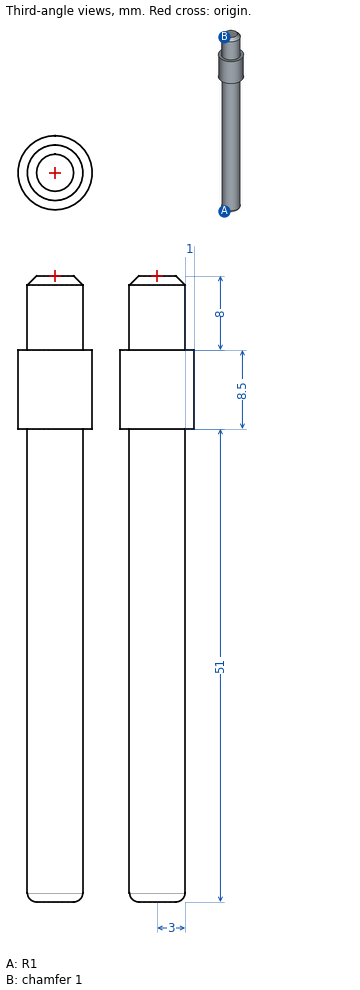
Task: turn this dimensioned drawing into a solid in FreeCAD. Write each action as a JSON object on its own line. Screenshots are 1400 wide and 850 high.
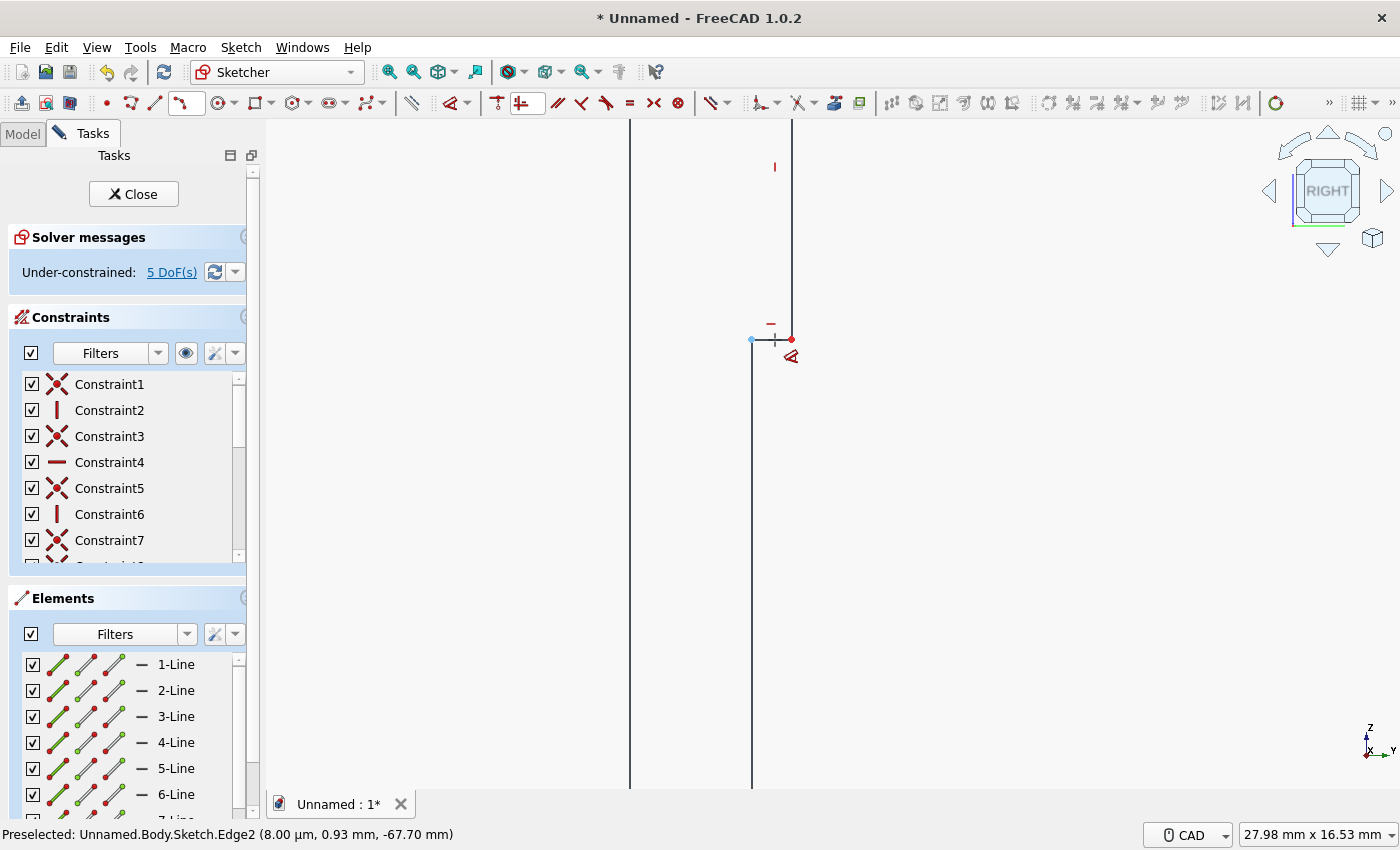
{"action": "left_click", "coordinate": [772, 340]}
{"action": "left_click", "coordinate": [772, 306]}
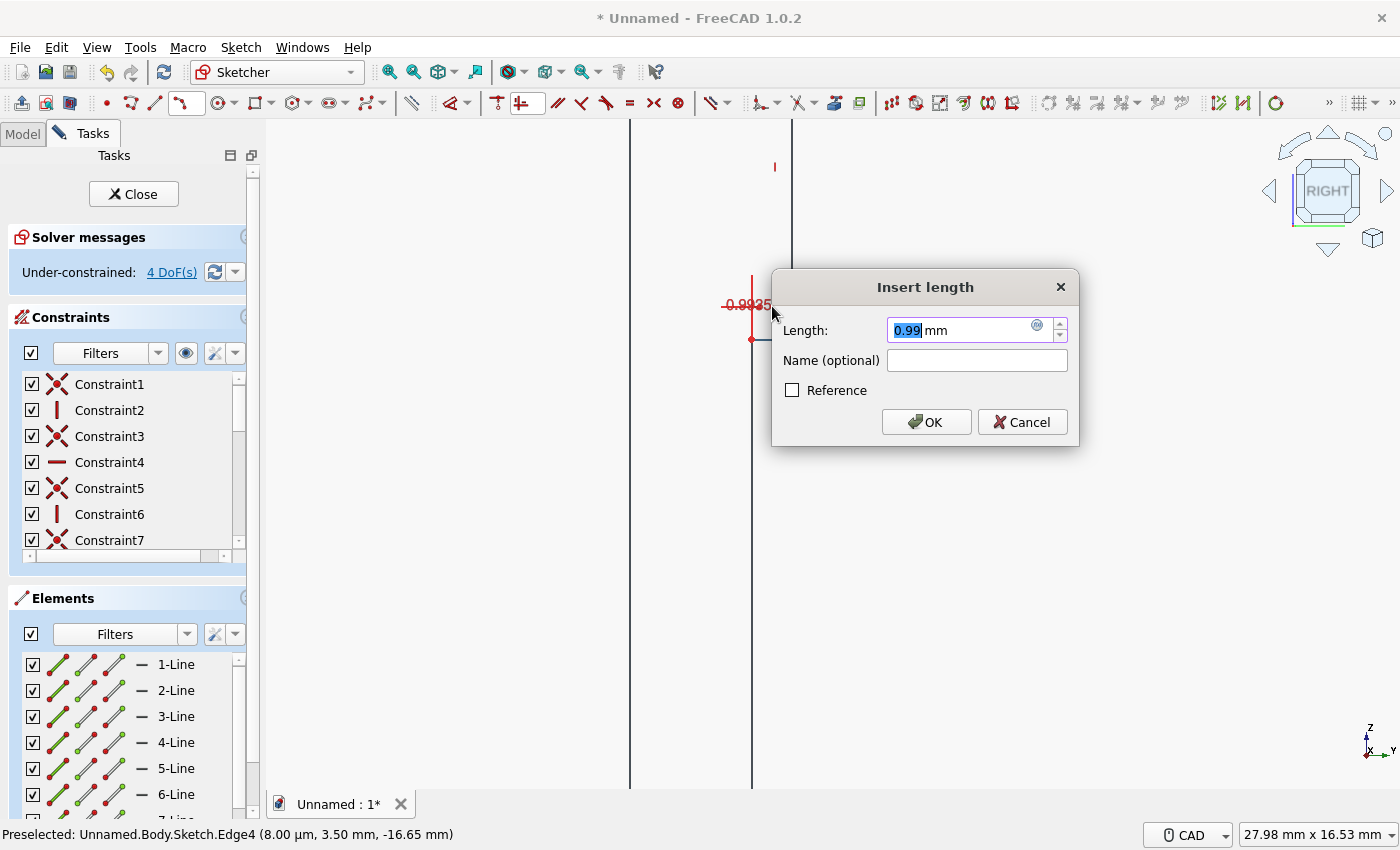
{"action": "type", "text": "1"}
{"action": "key", "text": "Return"}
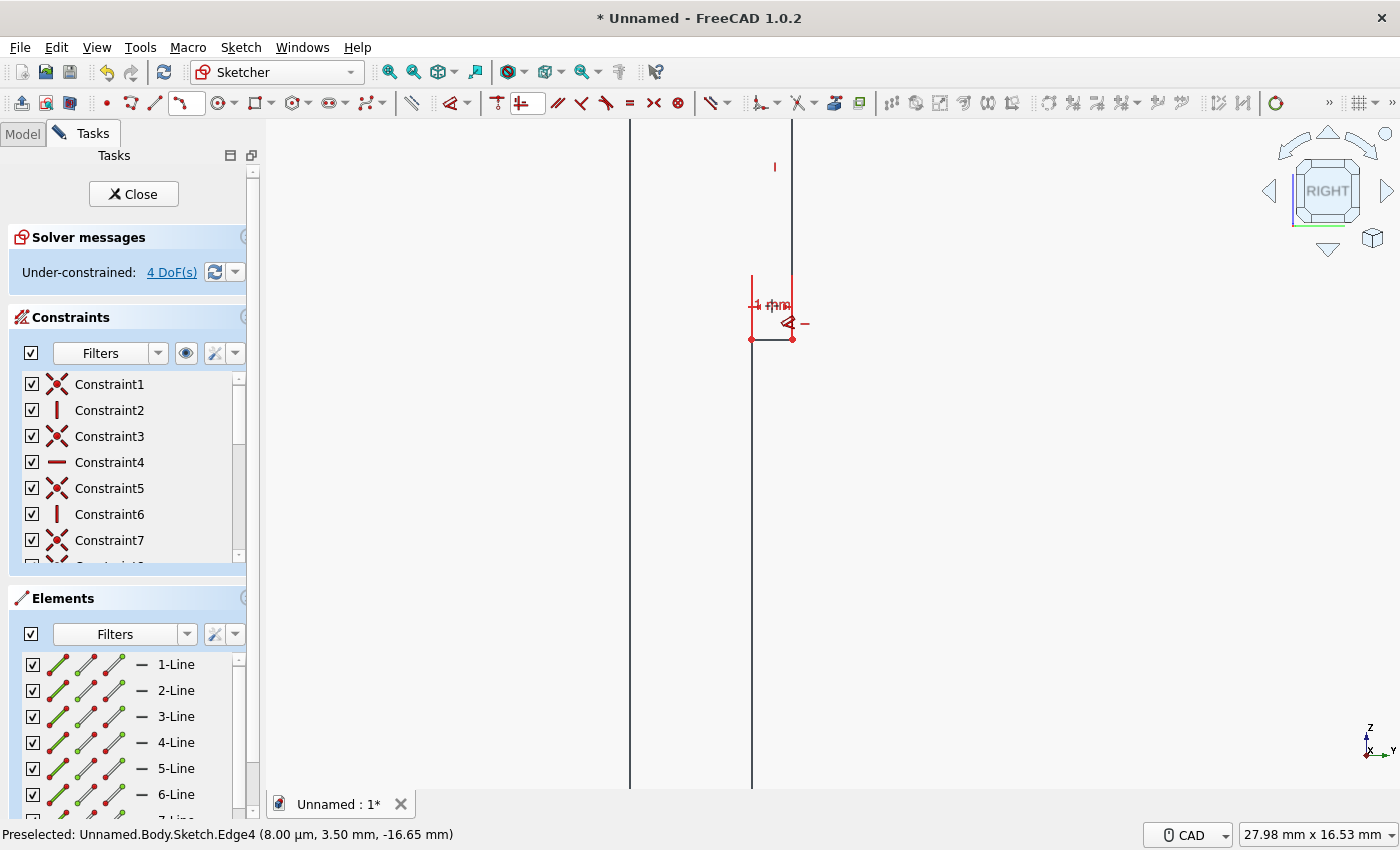
{"action": "scroll", "coordinate": [775, 339], "scroll_direction": "down", "scroll_amount": 9}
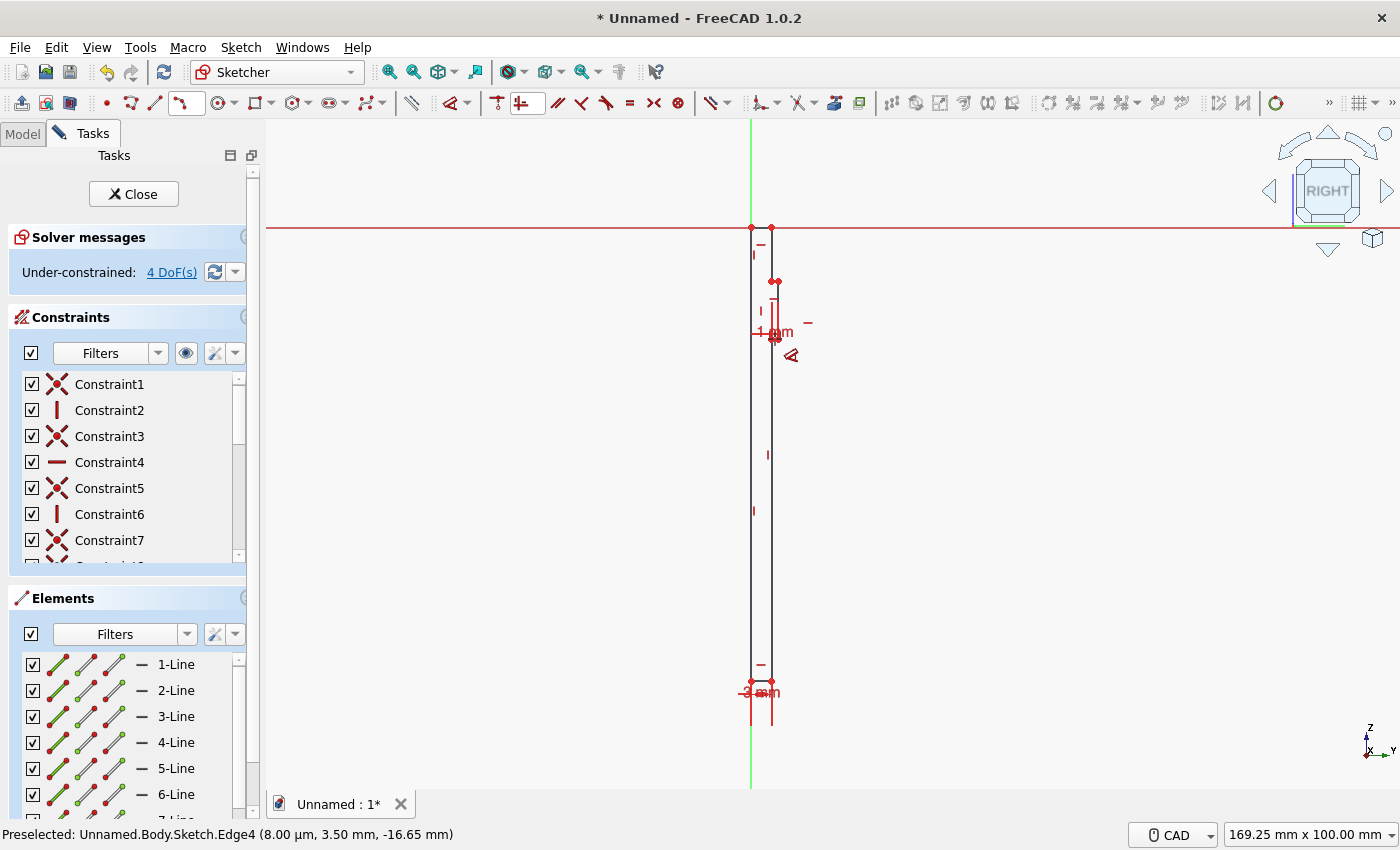
{"action": "scroll", "coordinate": [776, 282], "scroll_direction": "up", "scroll_amount": 10}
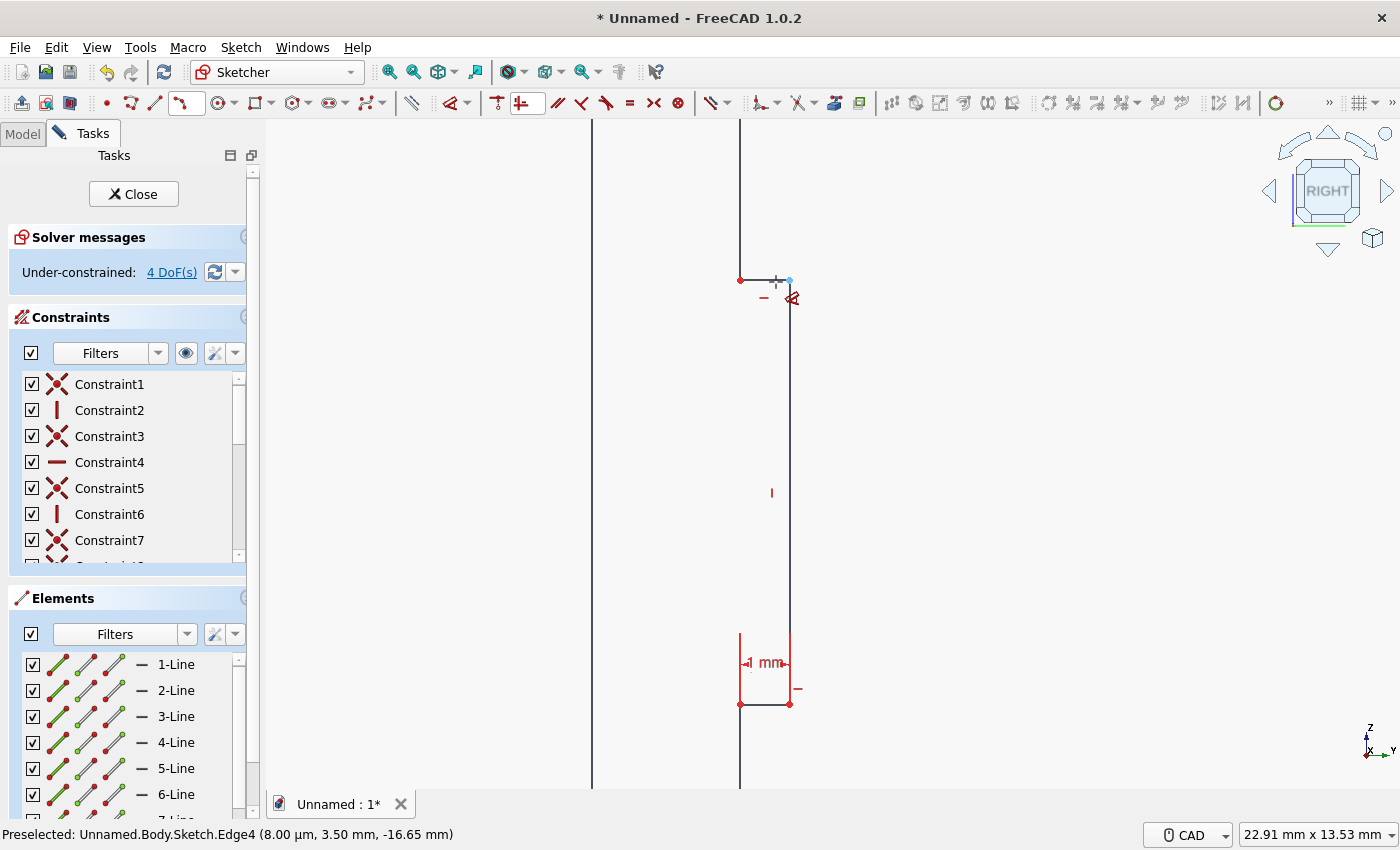
{"action": "left_click", "coordinate": [775, 280]}
{"action": "left_click", "coordinate": [765, 246]}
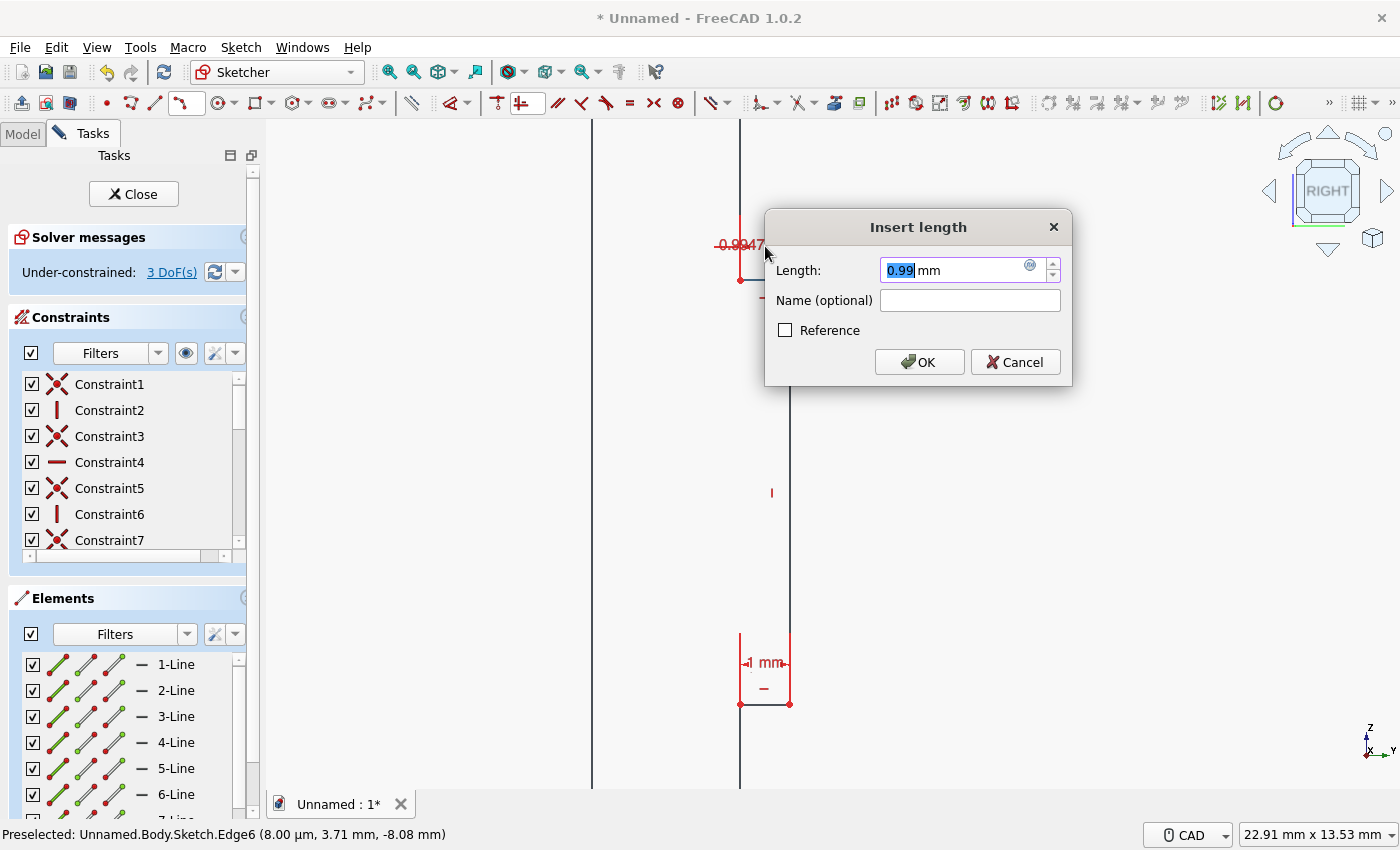
{"action": "type", "text": "1"}
{"action": "key", "text": "Return"}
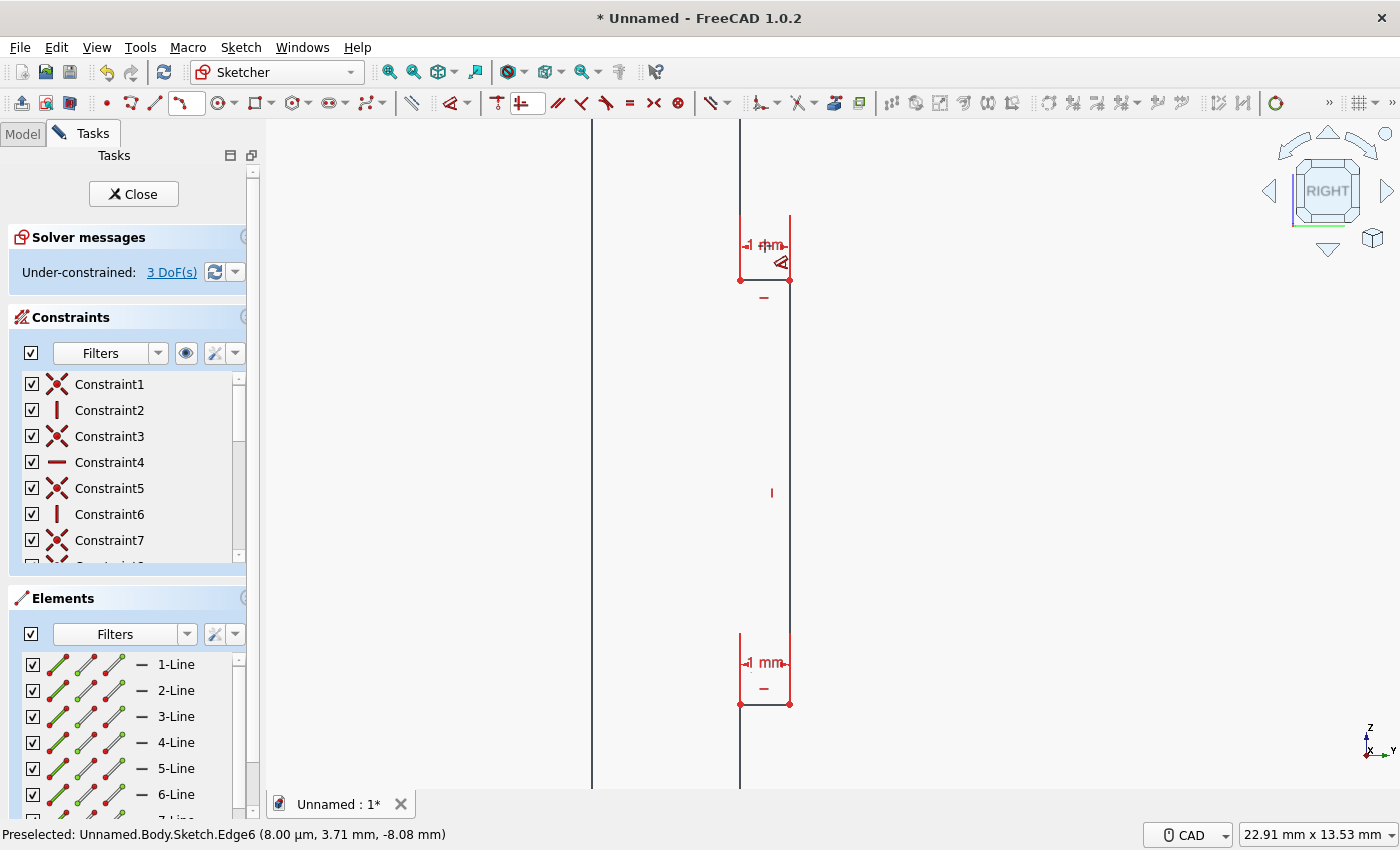
{"action": "scroll", "coordinate": [776, 282], "scroll_direction": "down", "scroll_amount": 10}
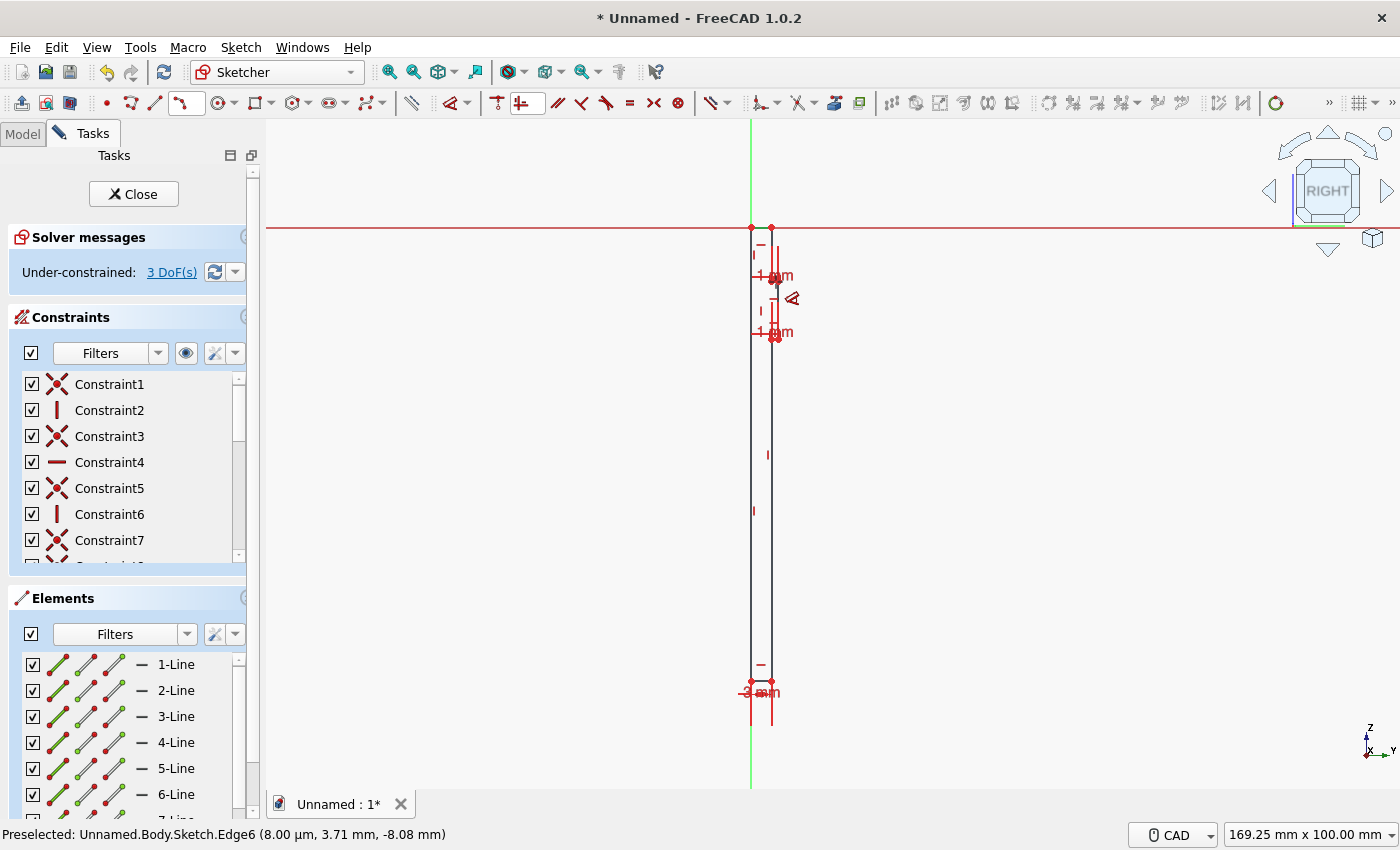
{"action": "left_click", "coordinate": [772, 266]}
{"action": "left_click", "coordinate": [806, 255]}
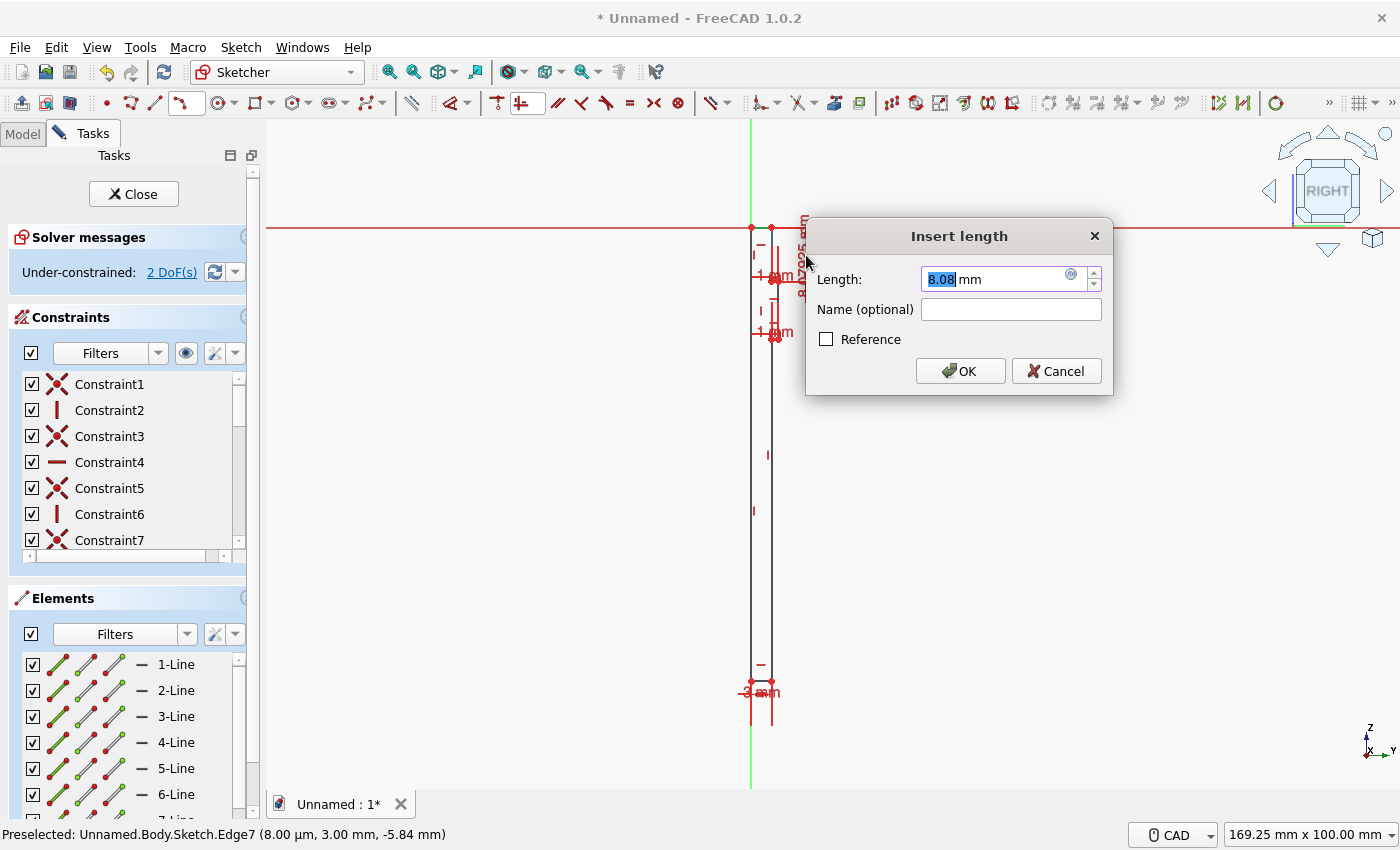
{"action": "type", "text": "8"}
{"action": "key", "text": "Return"}